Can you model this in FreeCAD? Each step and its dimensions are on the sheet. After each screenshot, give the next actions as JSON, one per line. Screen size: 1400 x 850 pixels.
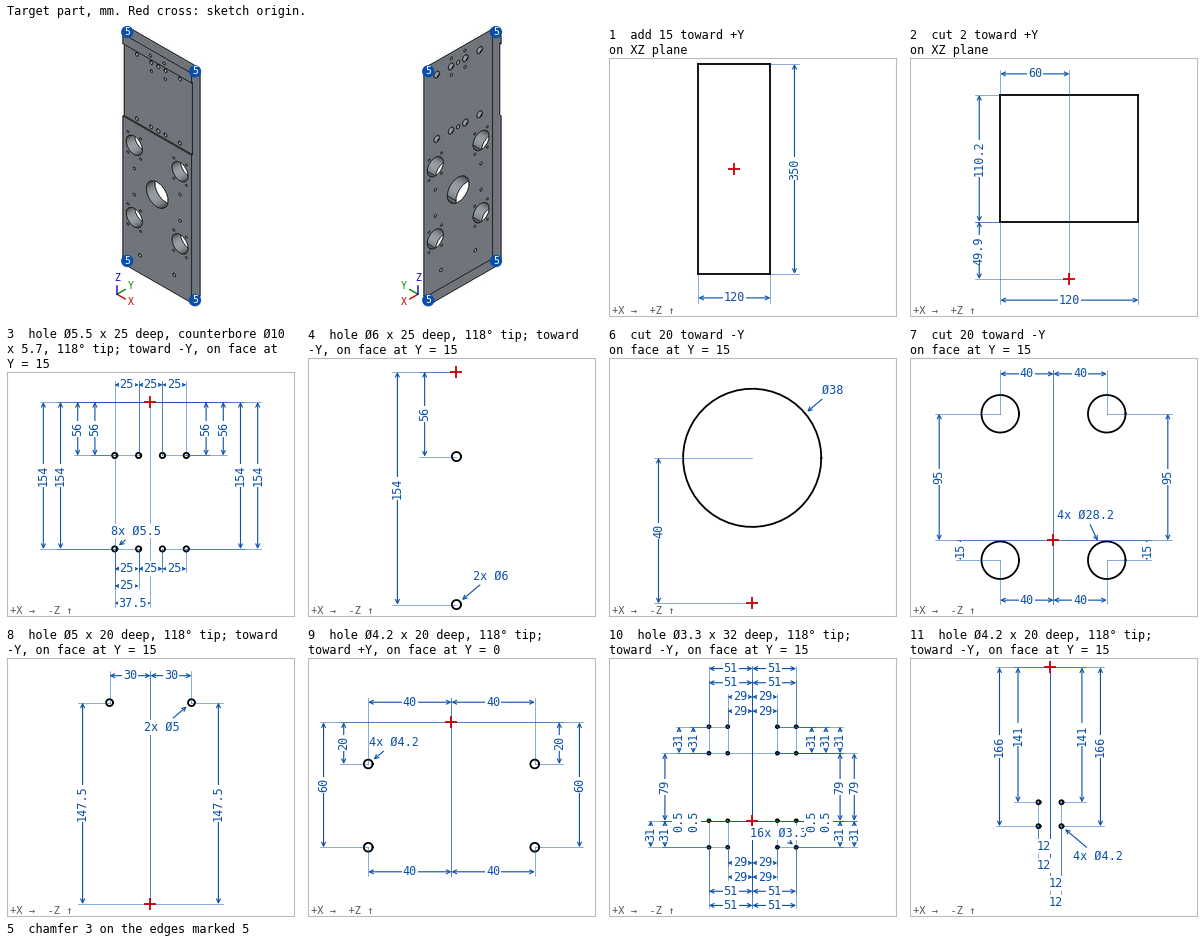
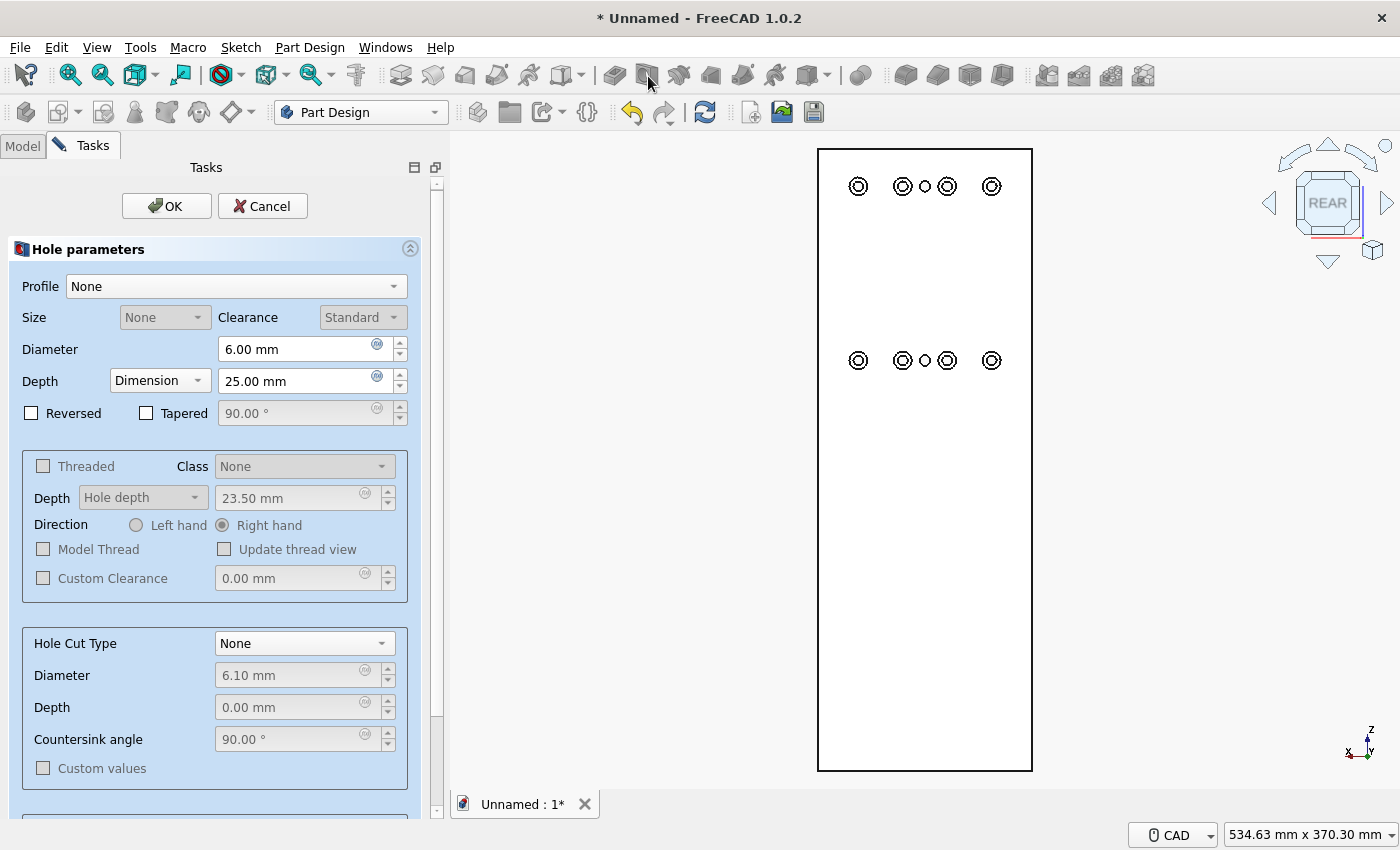
{"action": "triple_click", "coordinate": [305, 349]}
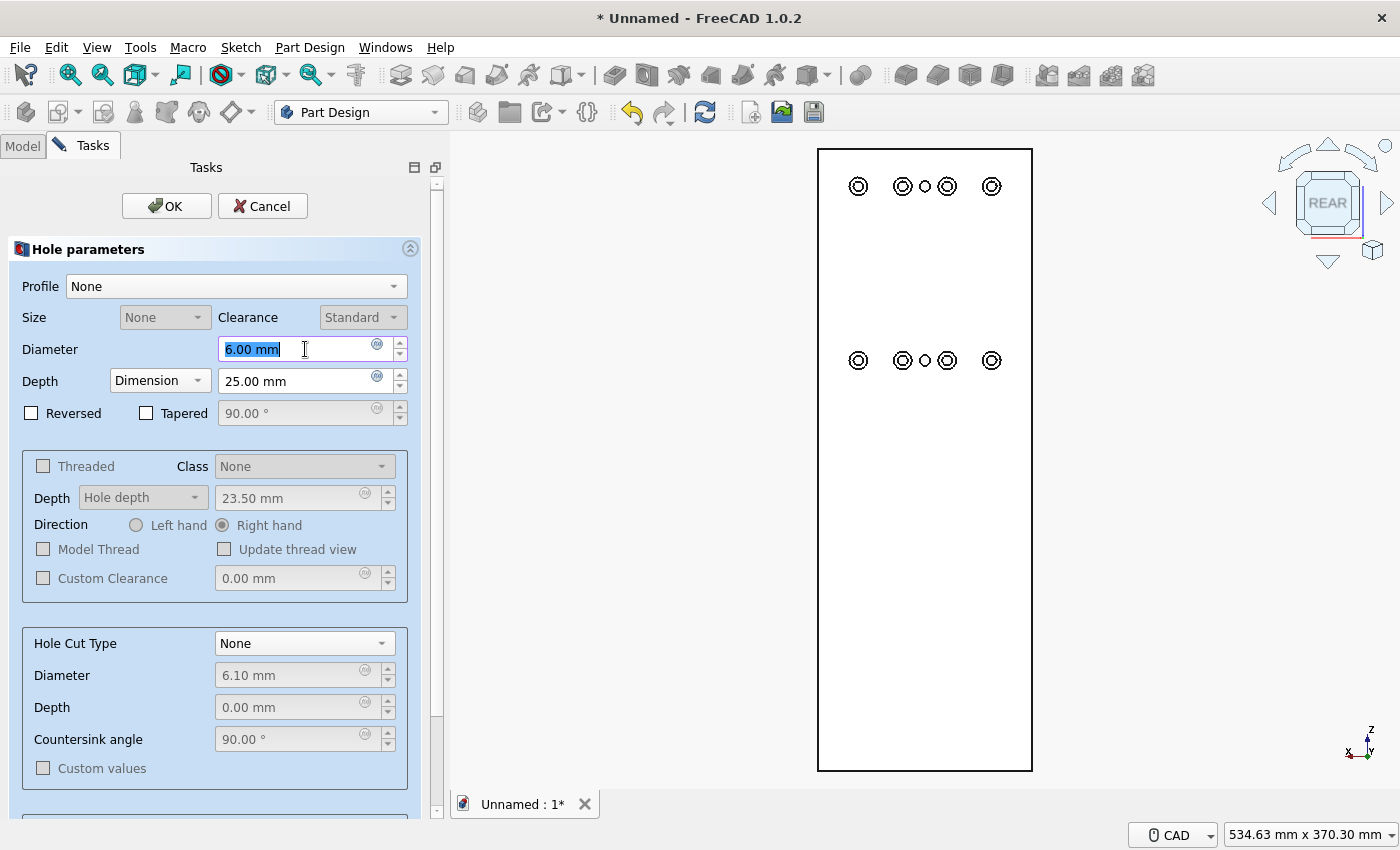
{"action": "type", "text": "6"}
{"action": "key", "text": "Tab"}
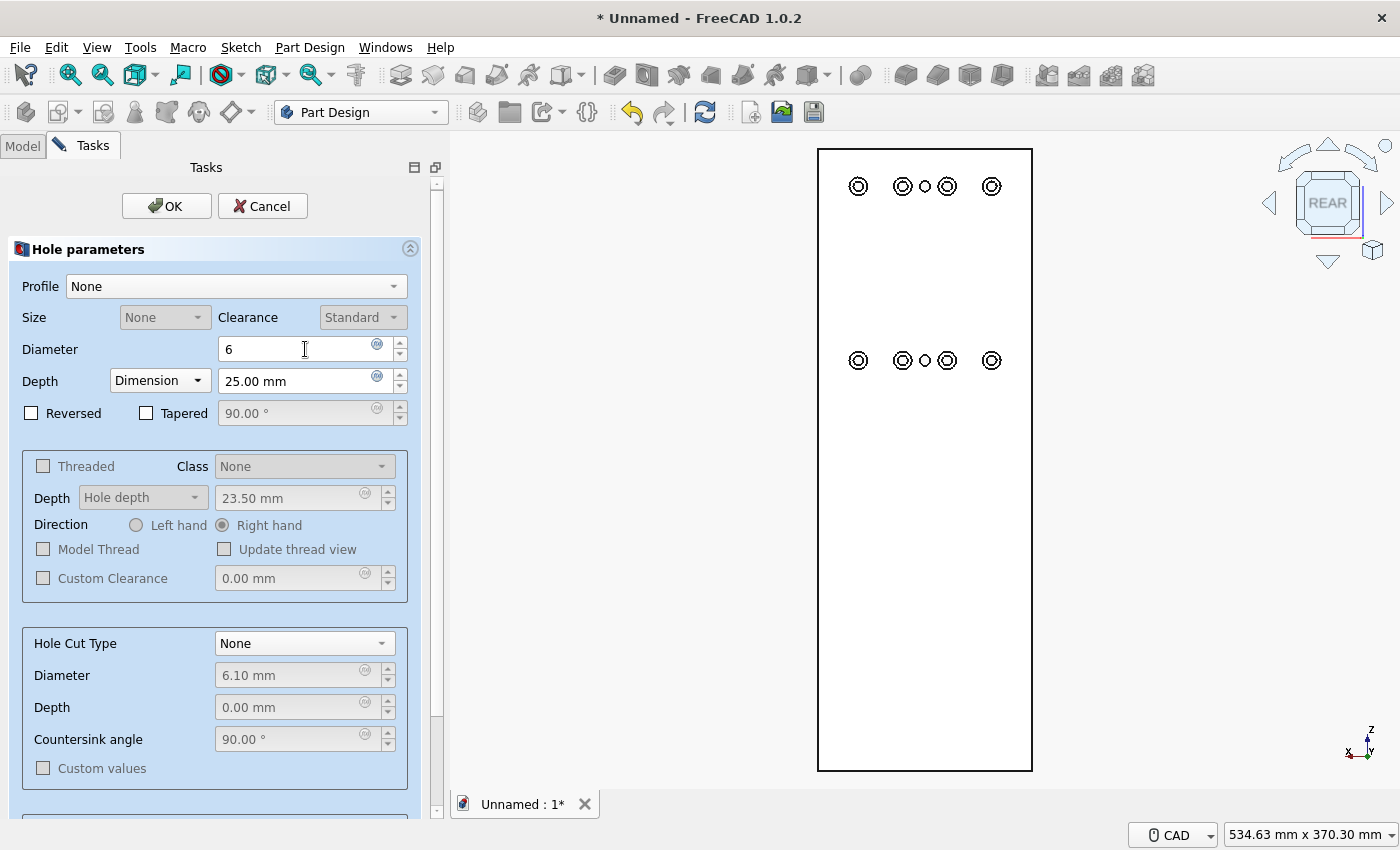
{"action": "triple_click", "coordinate": [305, 381]}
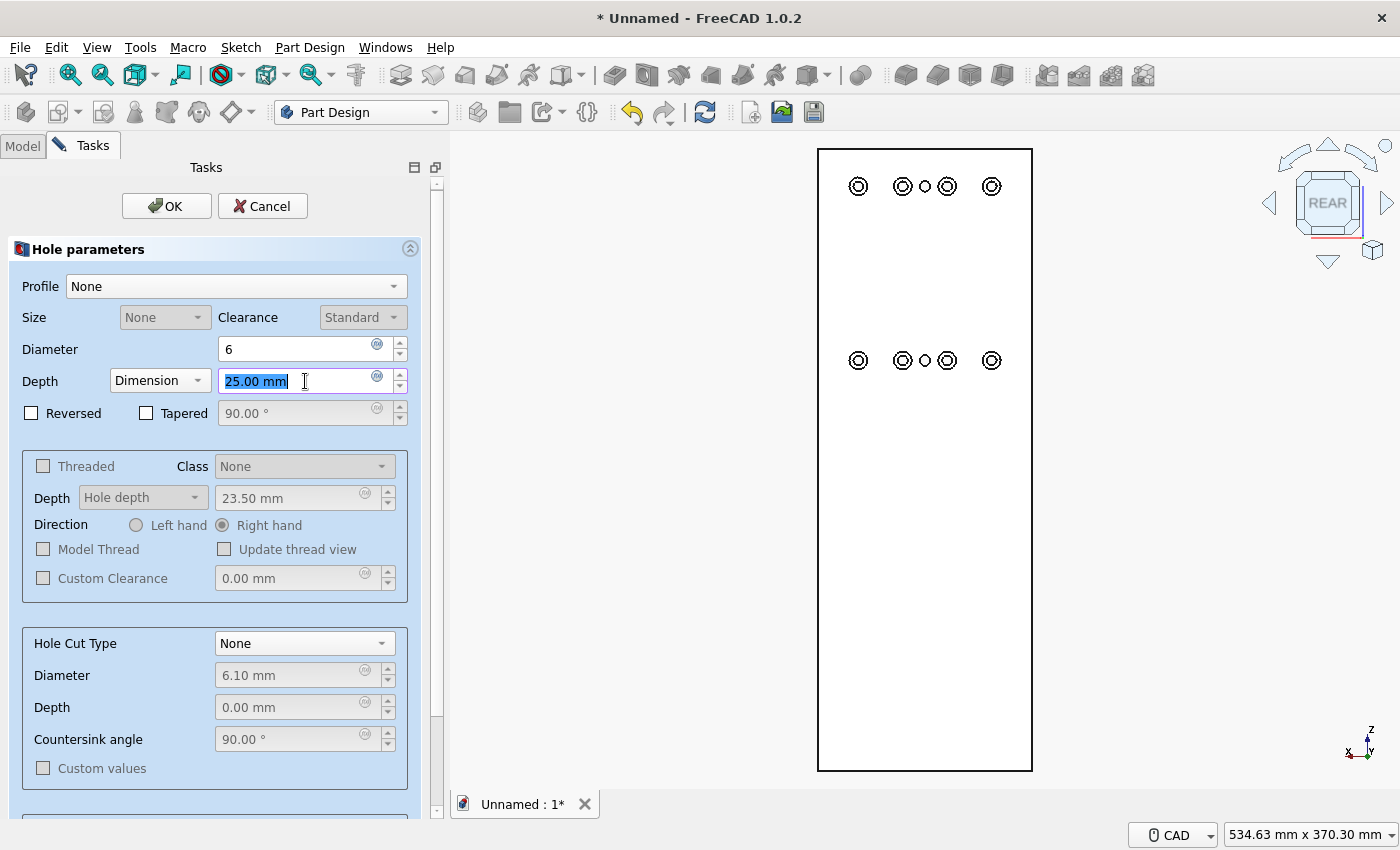
{"action": "type", "text": "25"}
{"action": "key", "text": "Tab"}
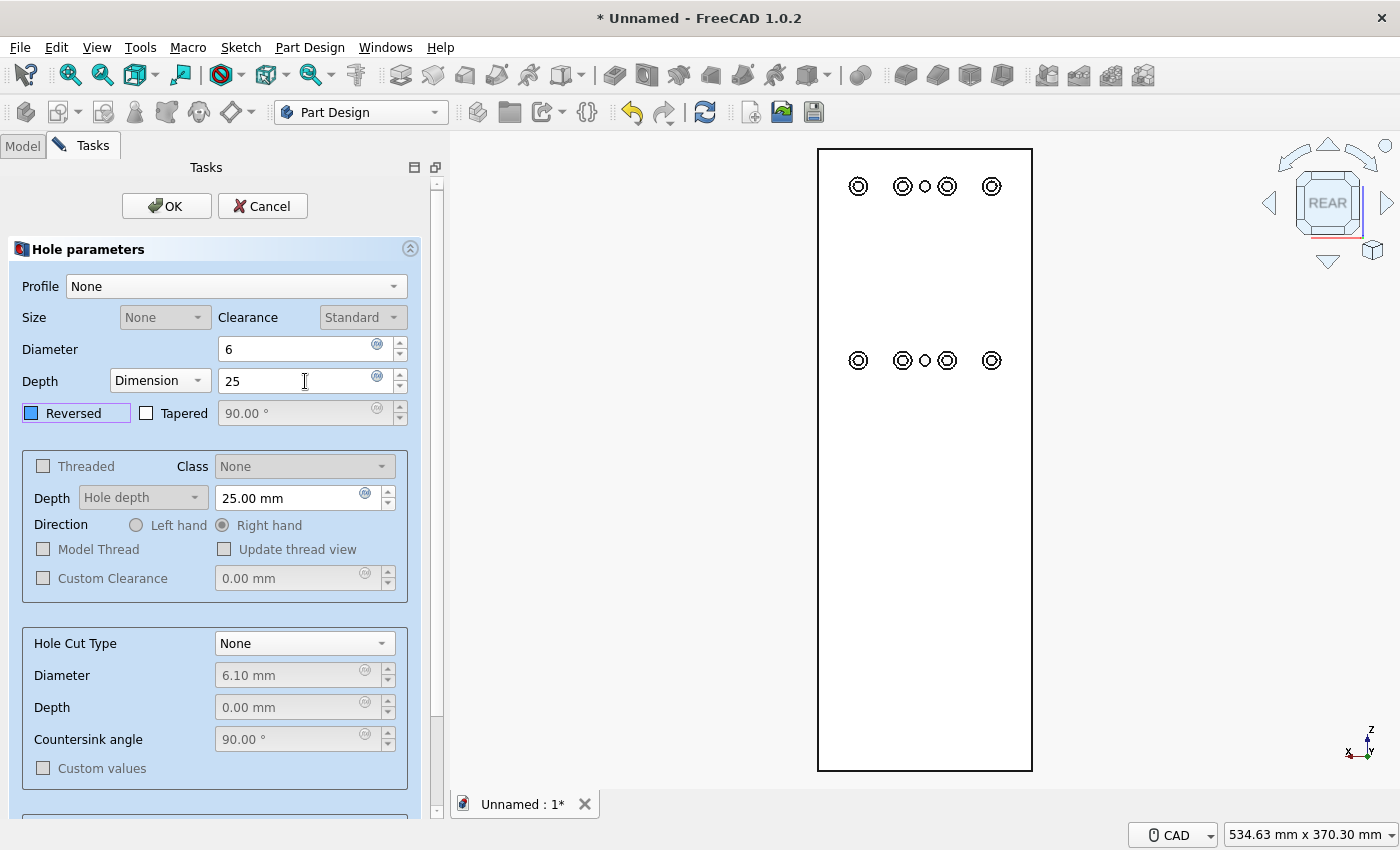
{"action": "left_click", "coordinate": [167, 206]}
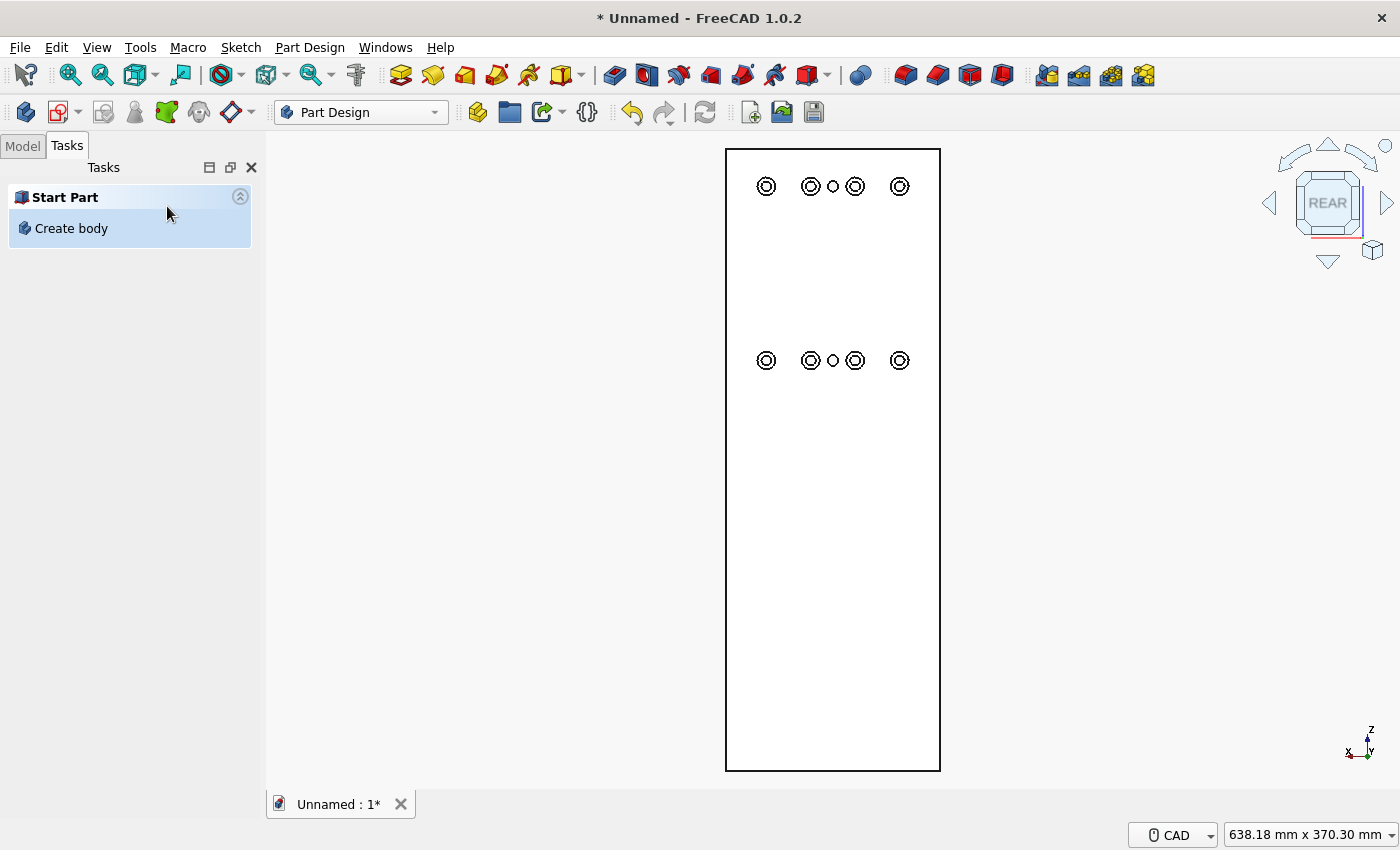
{"action": "key", "text": "0"}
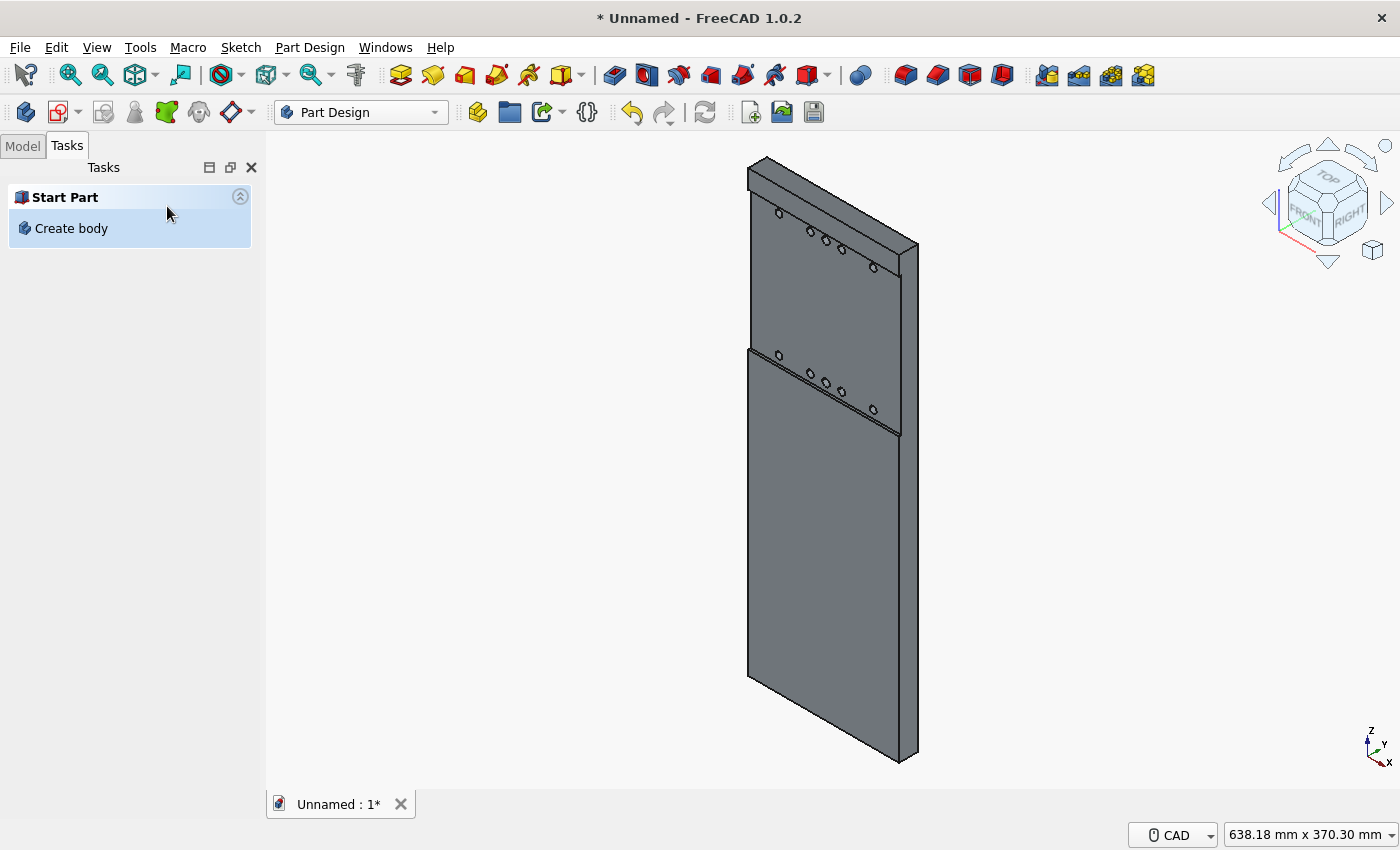
{"action": "left_click", "coordinate": [908, 249]}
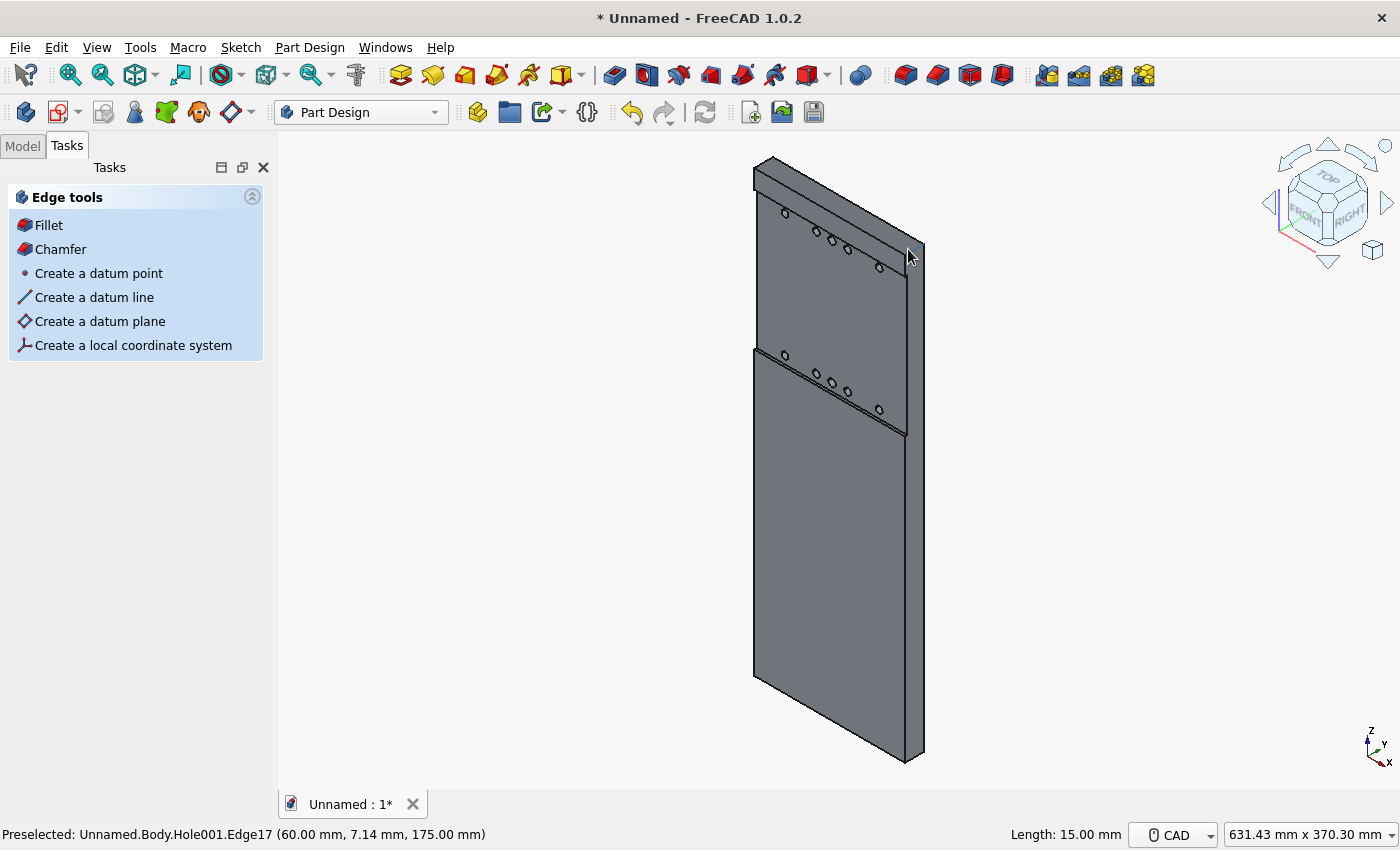
{"action": "key", "text": "2"}